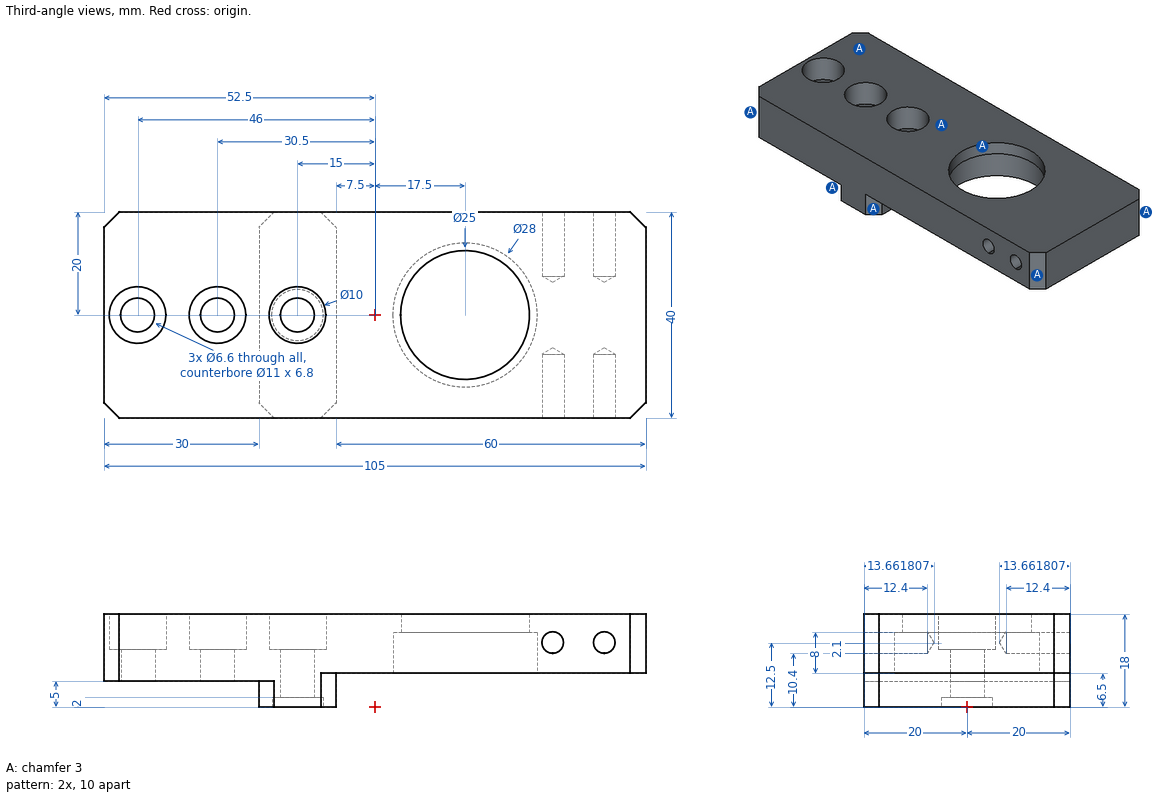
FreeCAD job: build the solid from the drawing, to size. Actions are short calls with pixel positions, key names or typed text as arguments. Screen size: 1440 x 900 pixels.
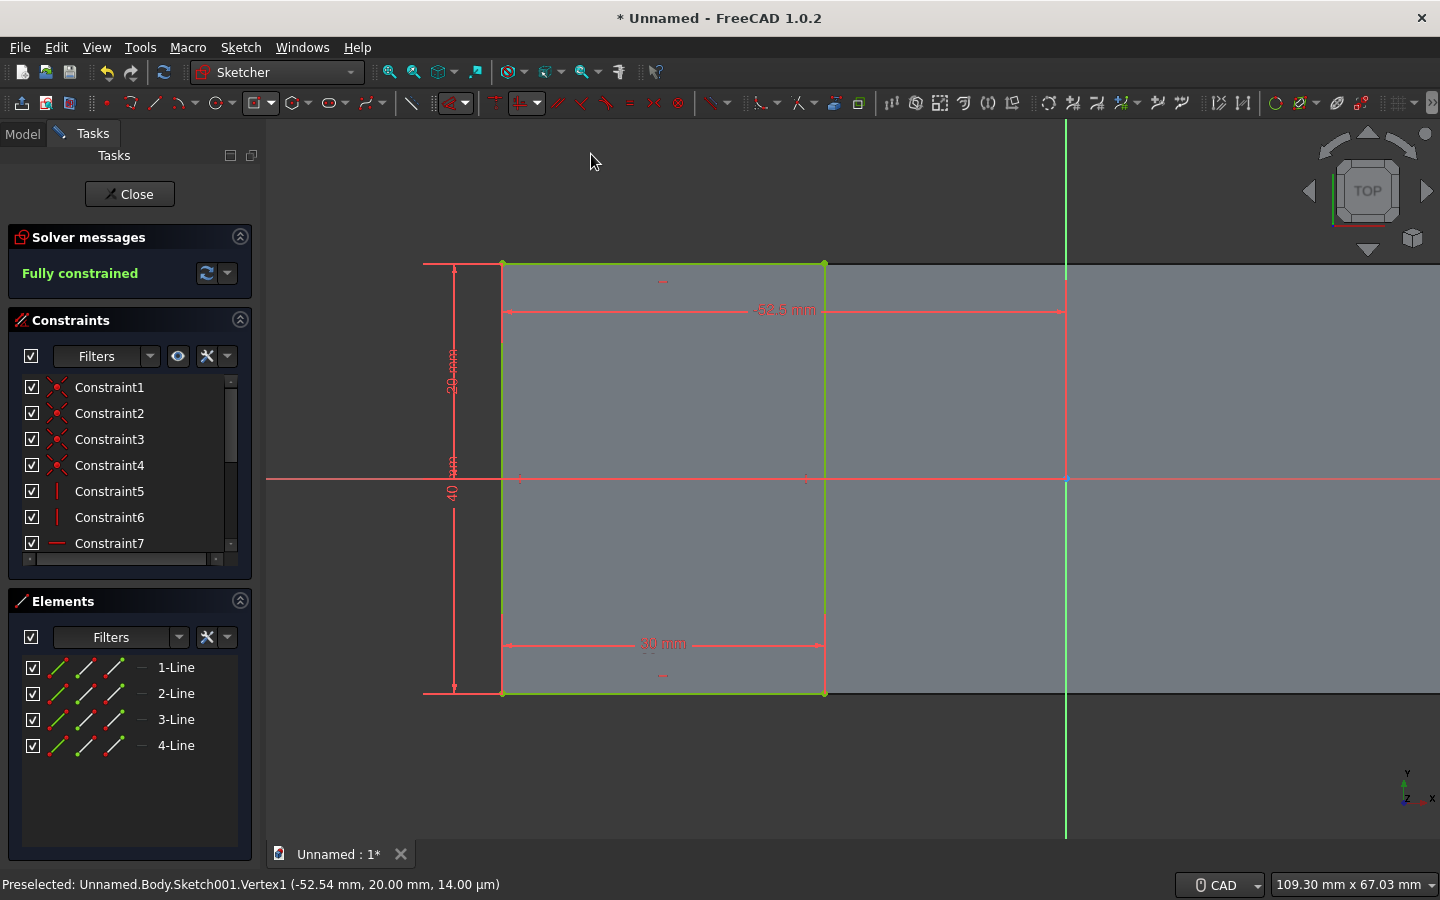
click(130, 194)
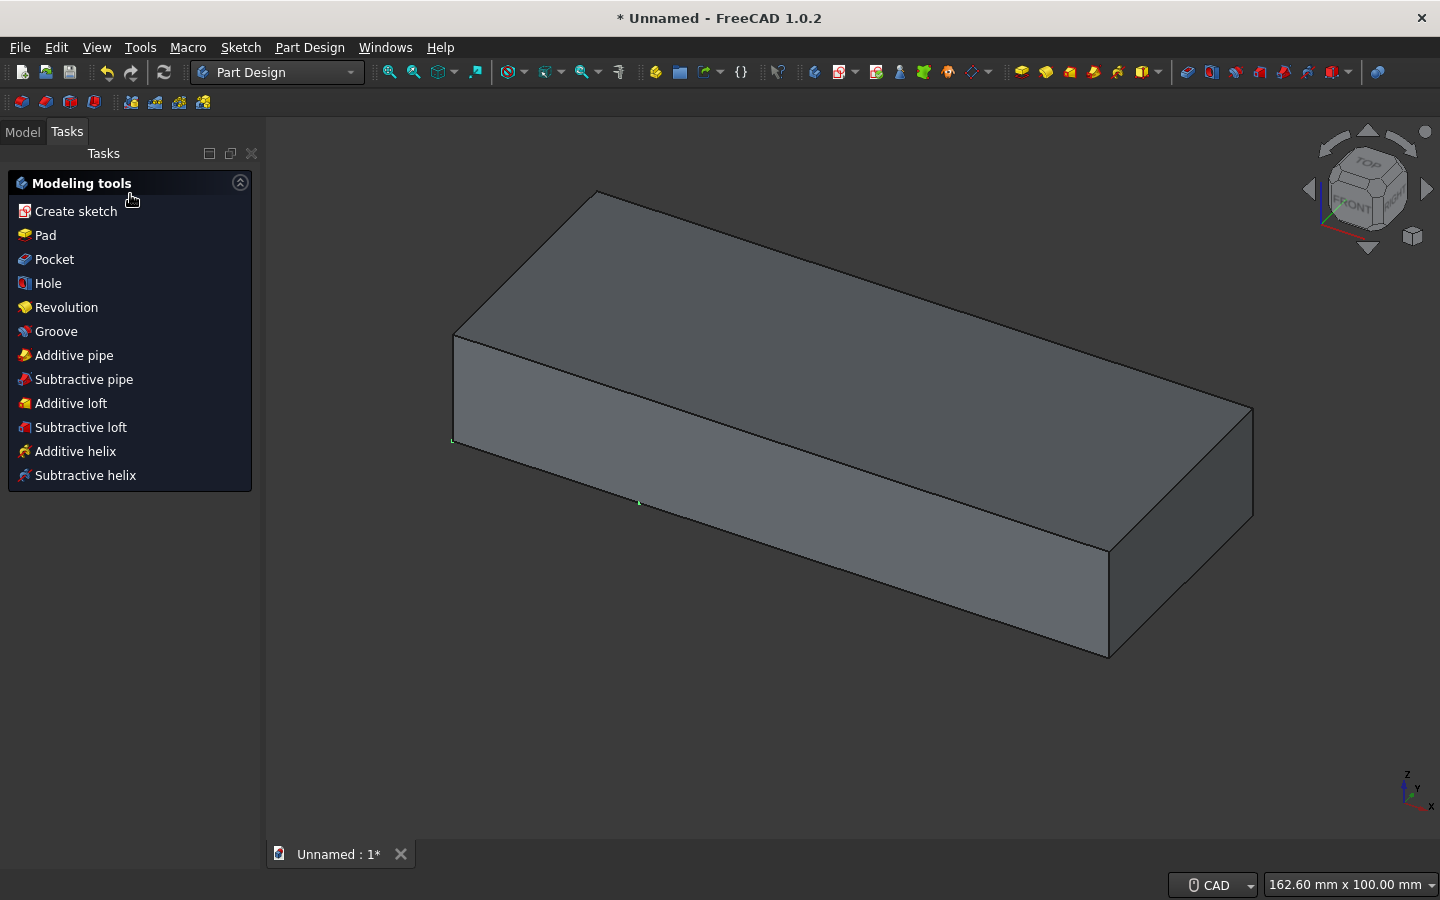
click(1188, 72)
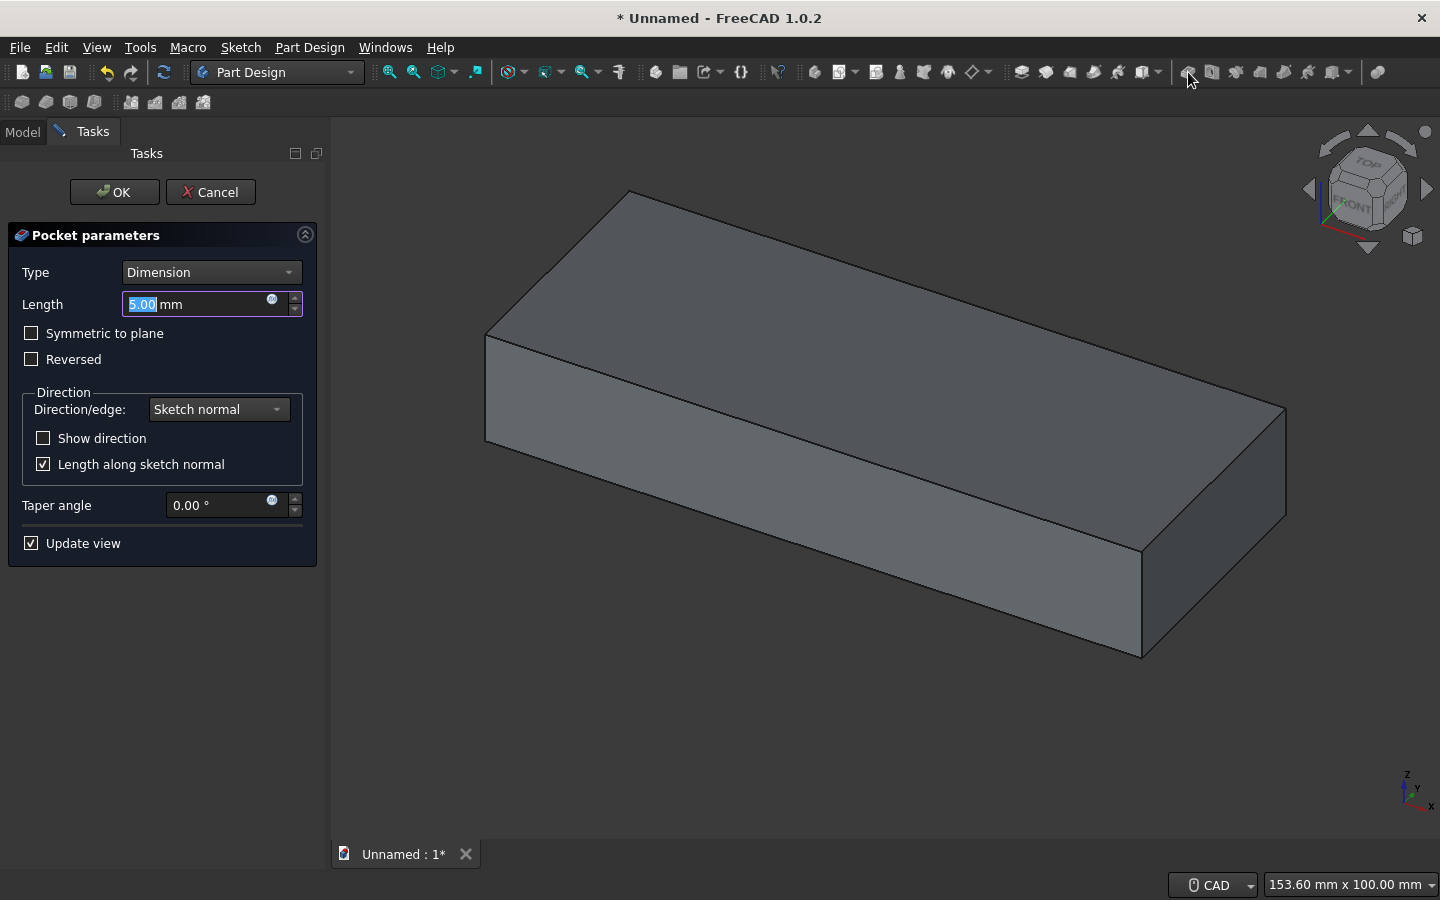
text(5)
key(Tab)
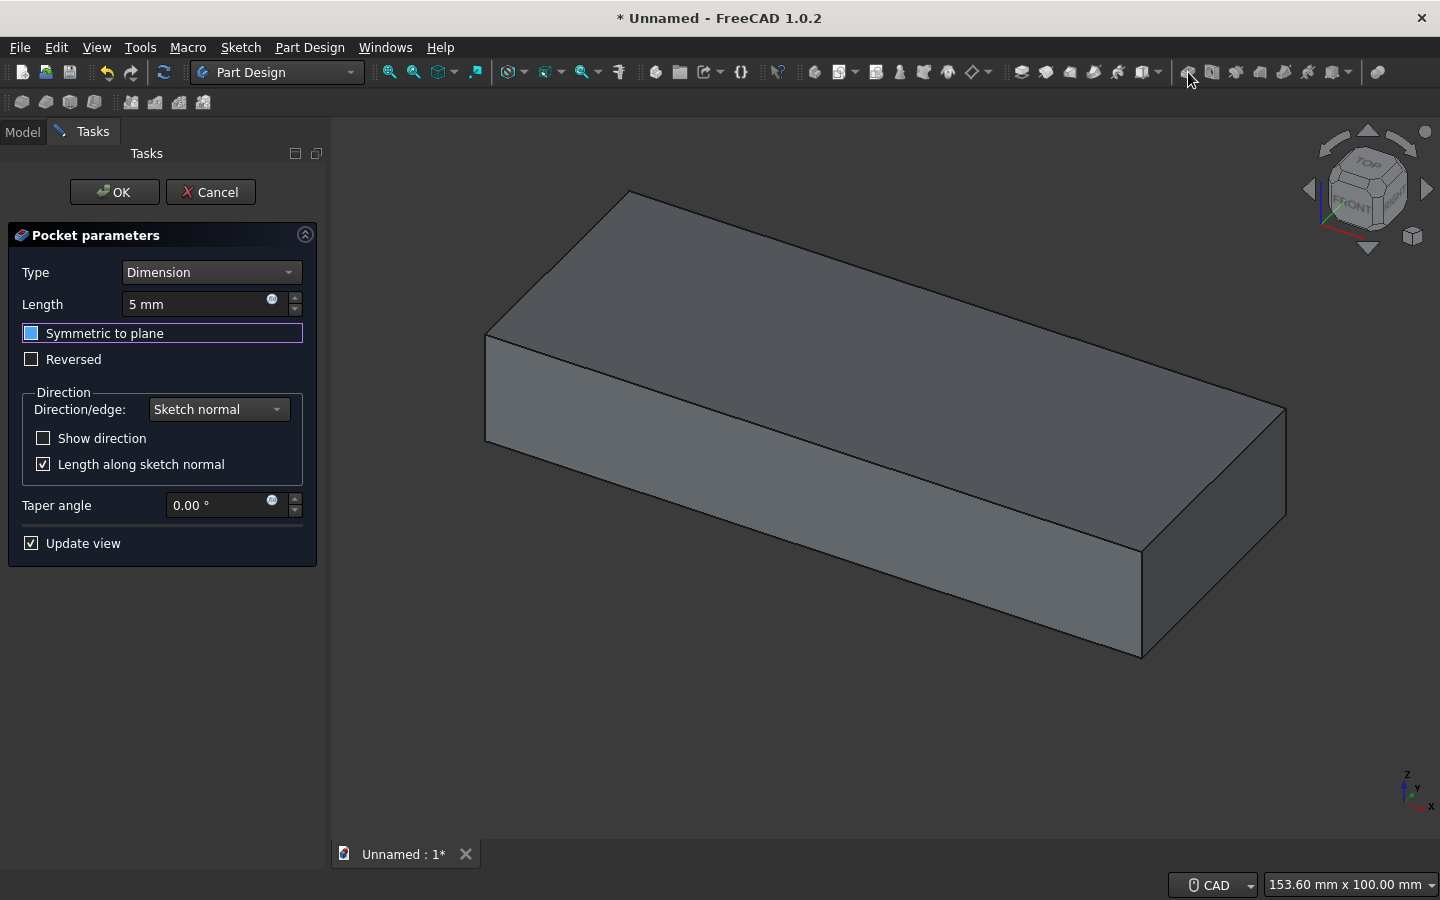
click(30, 359)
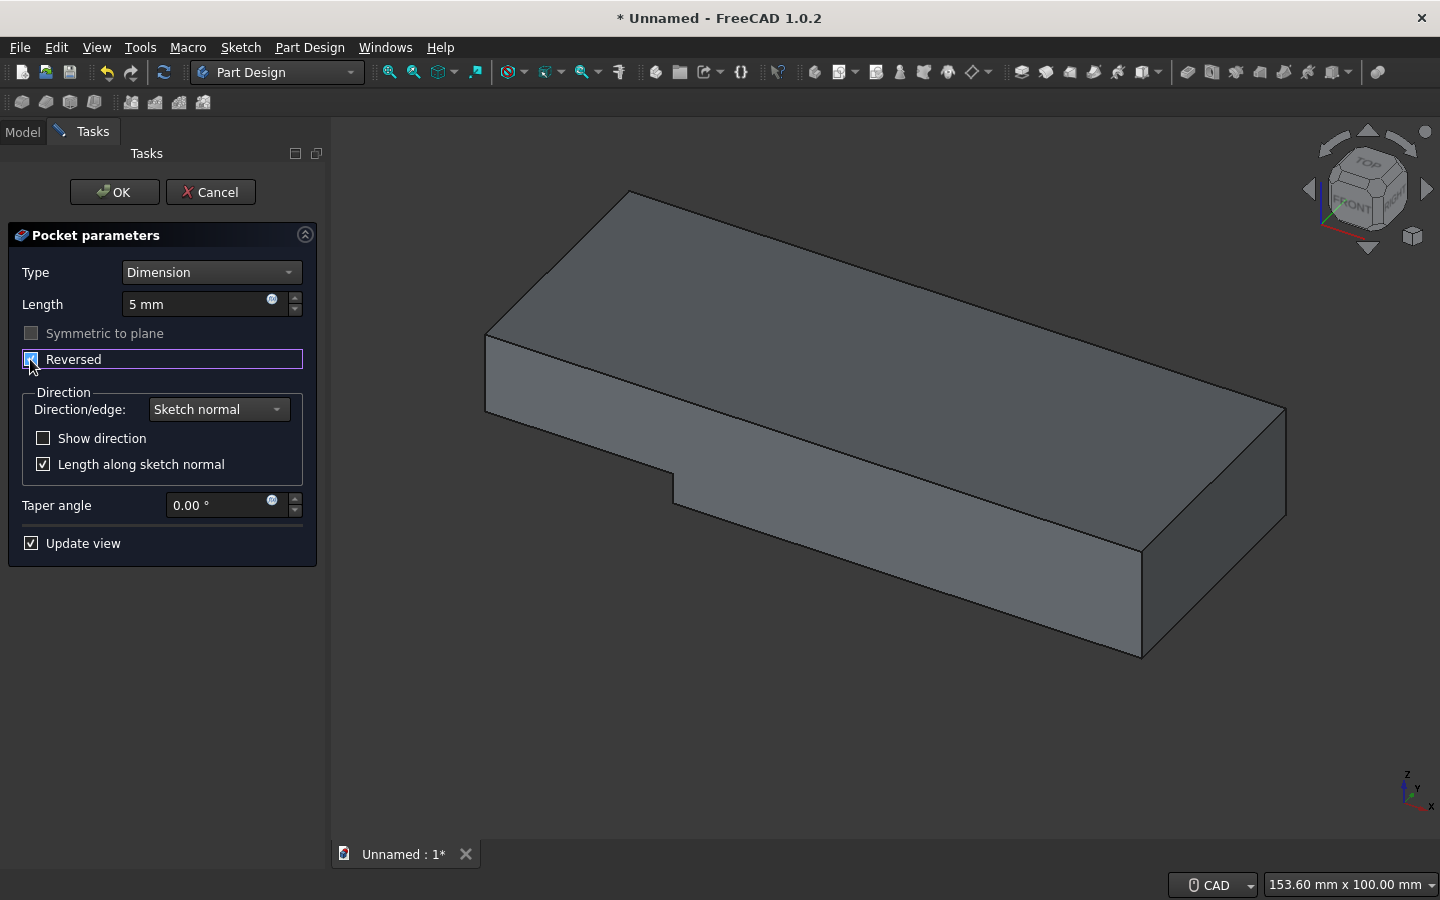
click(115, 192)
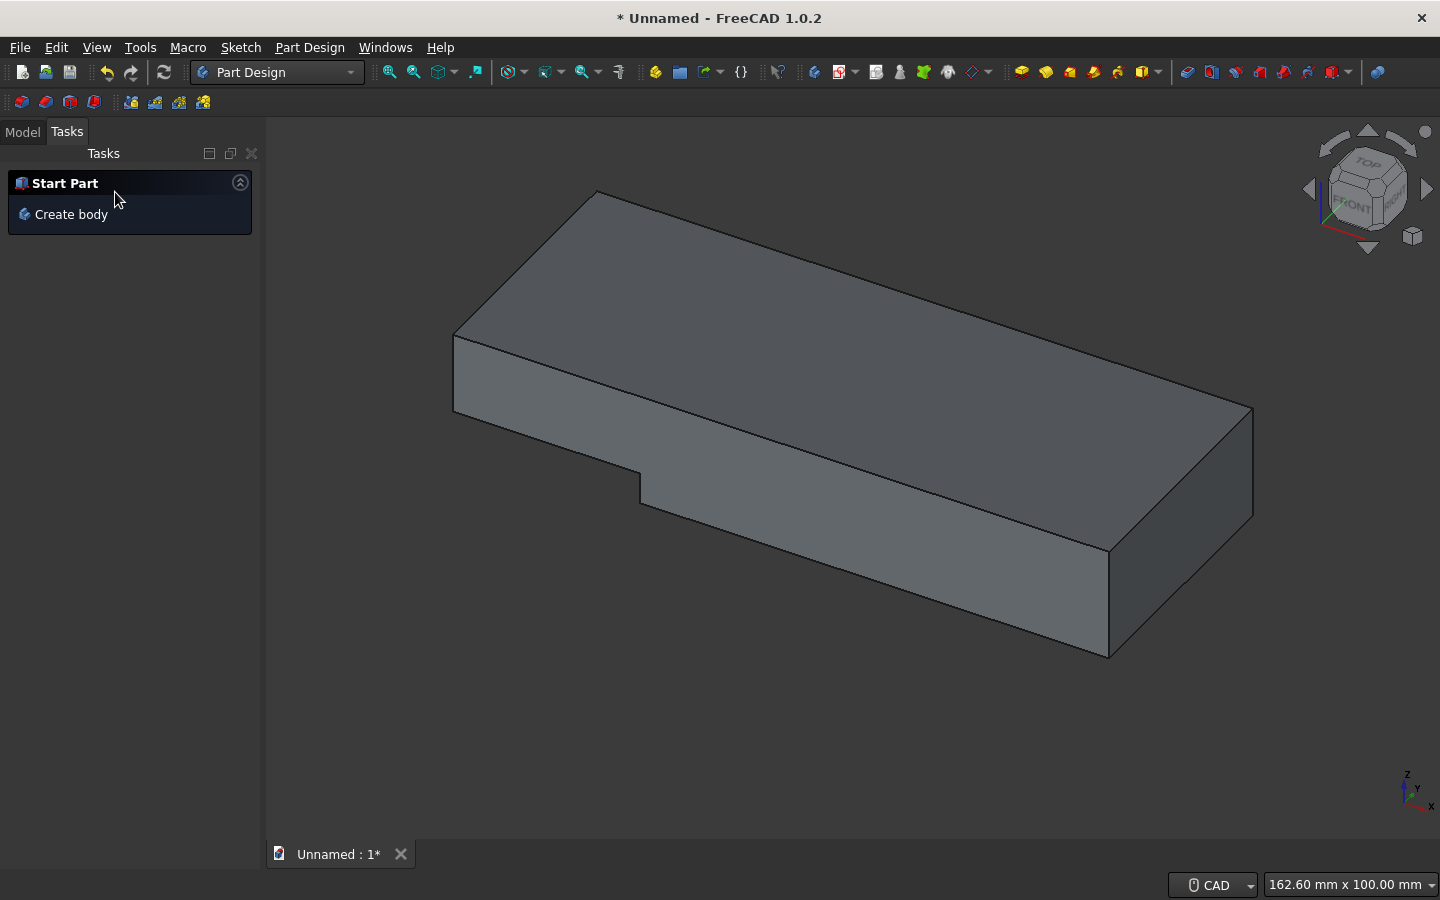
click(840, 72)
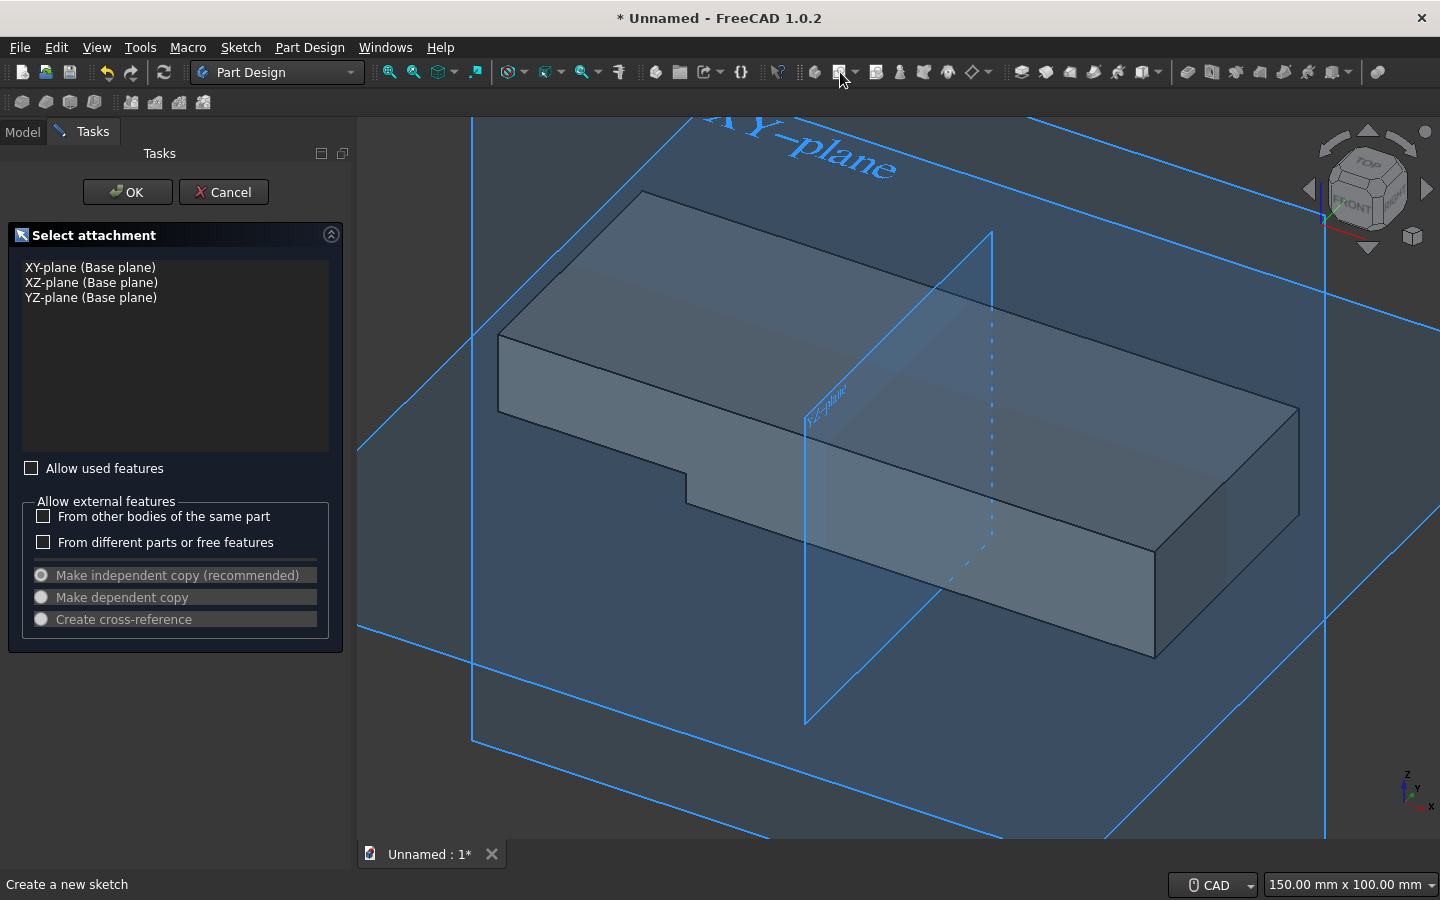
click(82, 268)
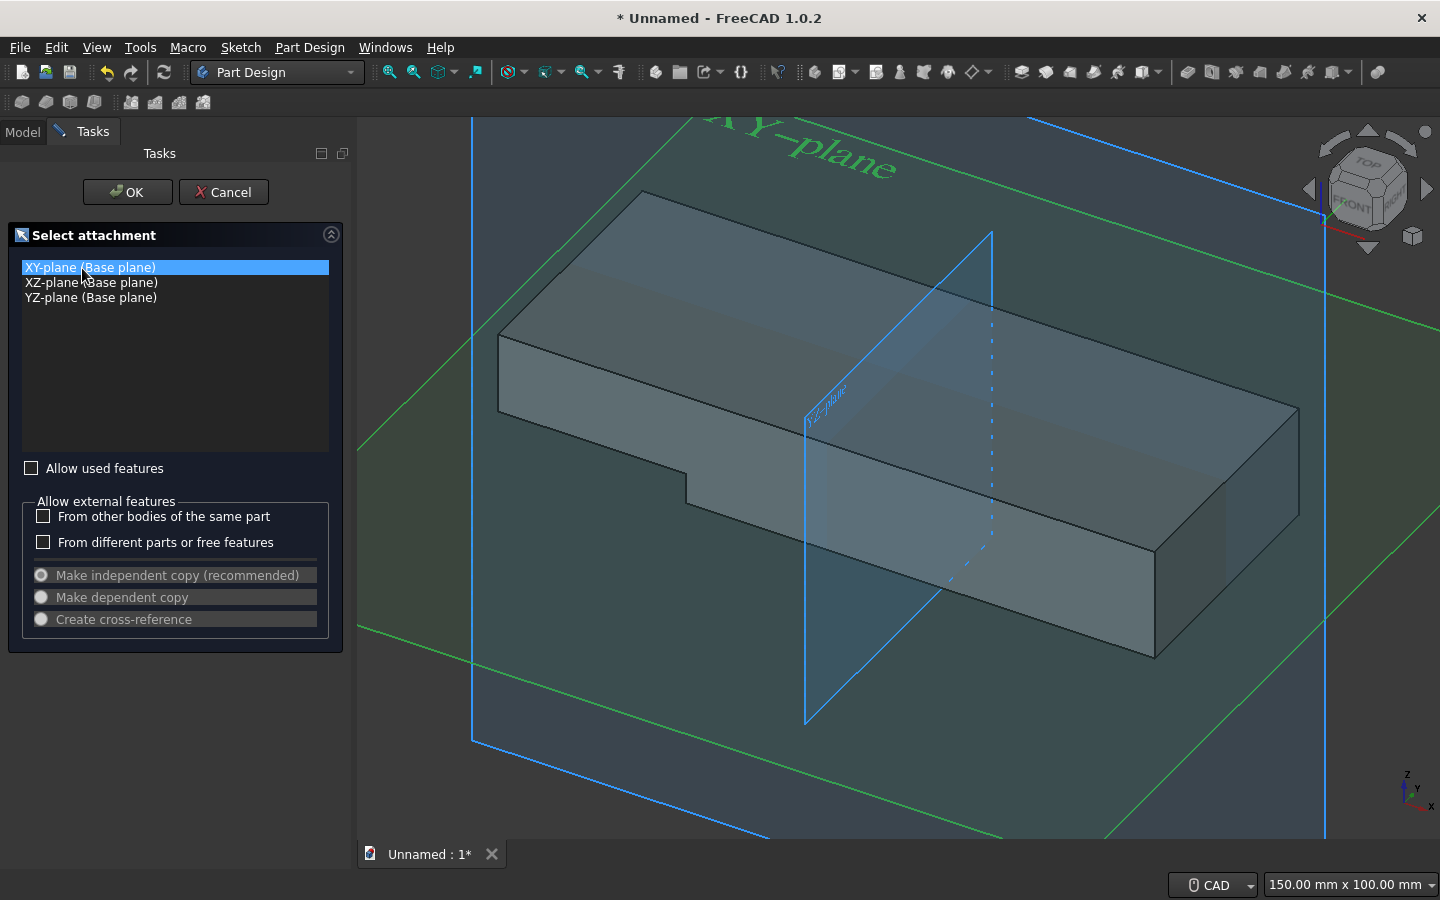
click(128, 192)